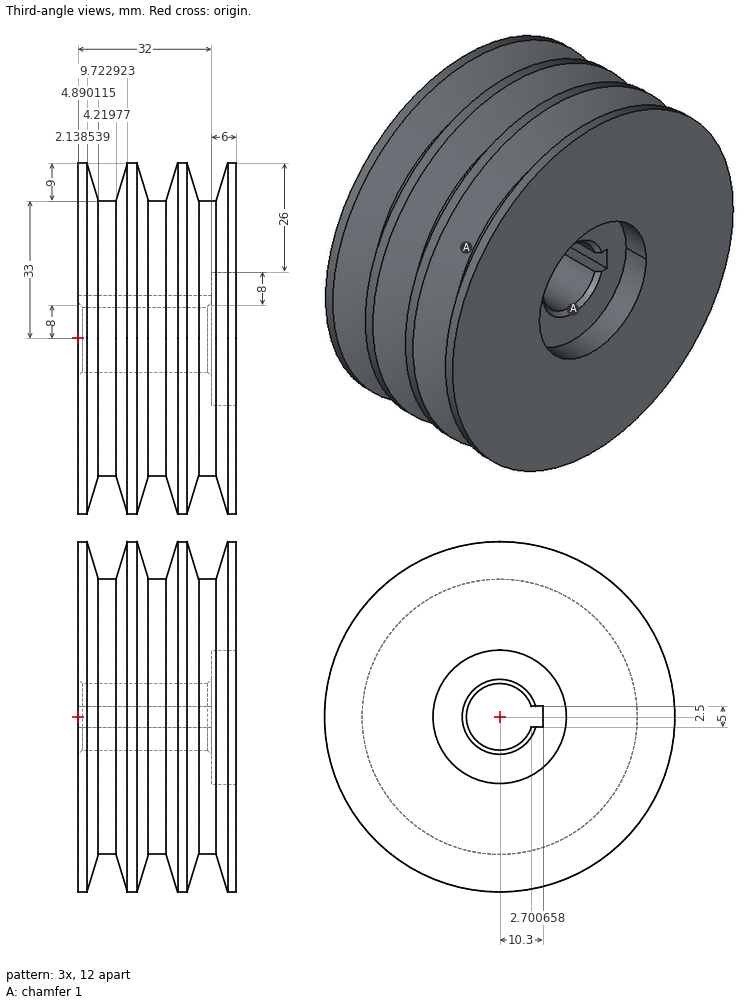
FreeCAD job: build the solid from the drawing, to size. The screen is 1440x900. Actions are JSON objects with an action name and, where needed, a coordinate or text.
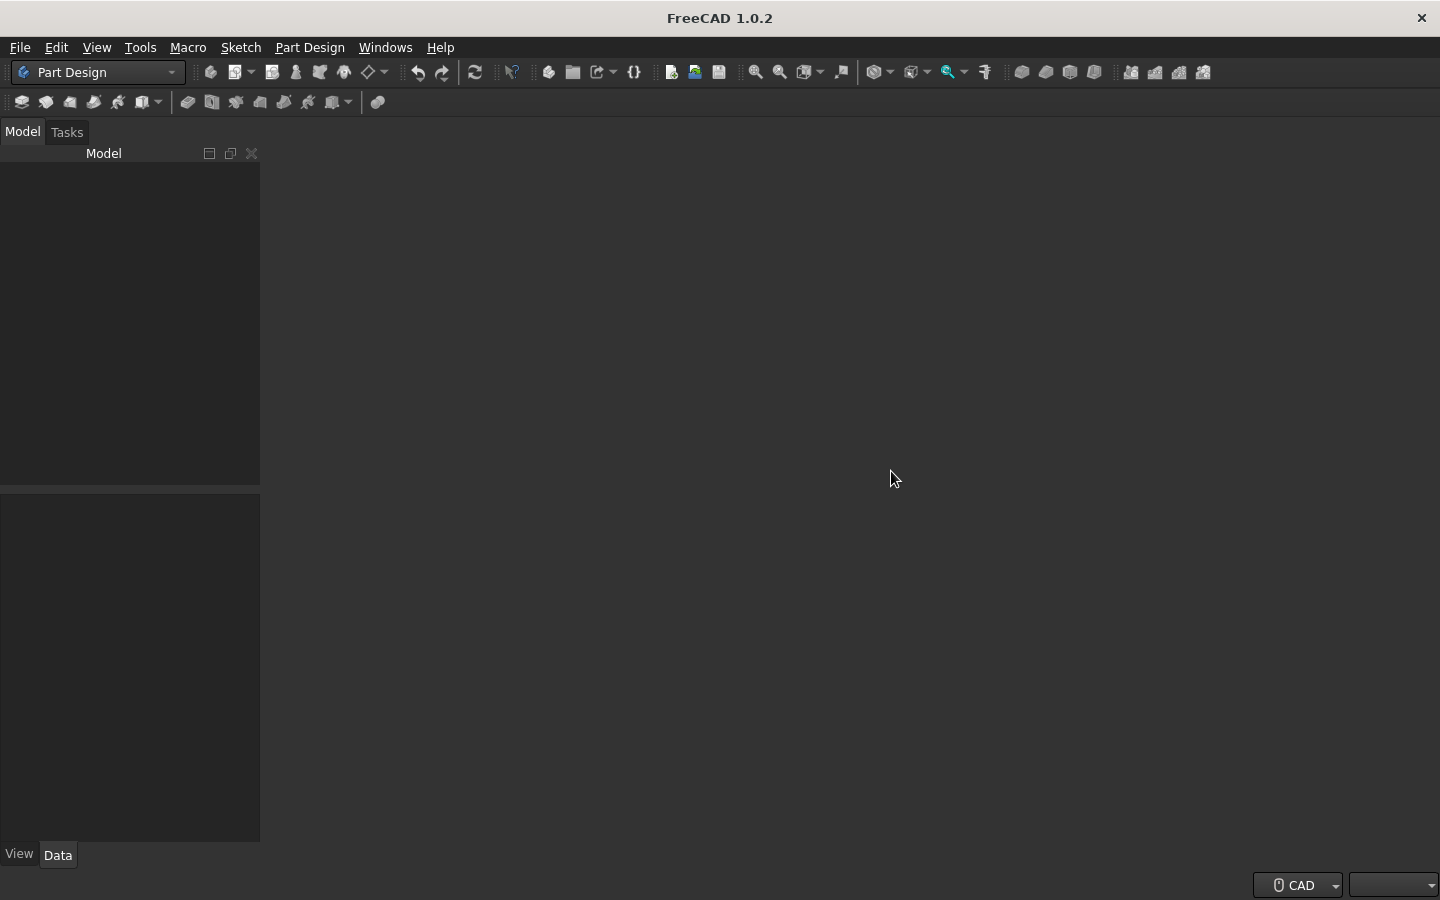
{"action": "key", "text": "ctrl+n"}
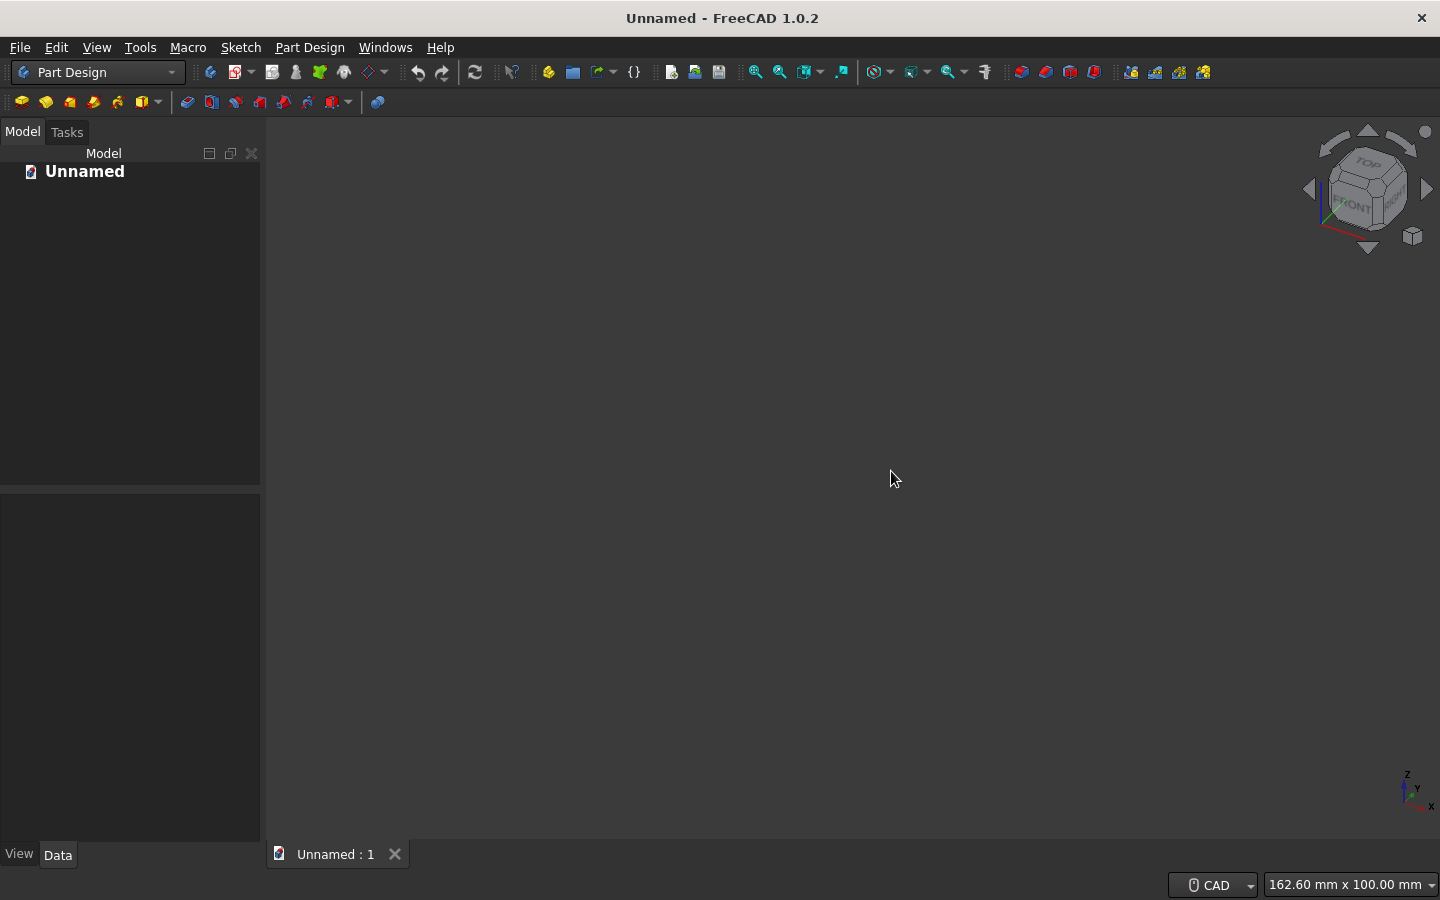
{"action": "left_click", "coordinate": [236, 72]}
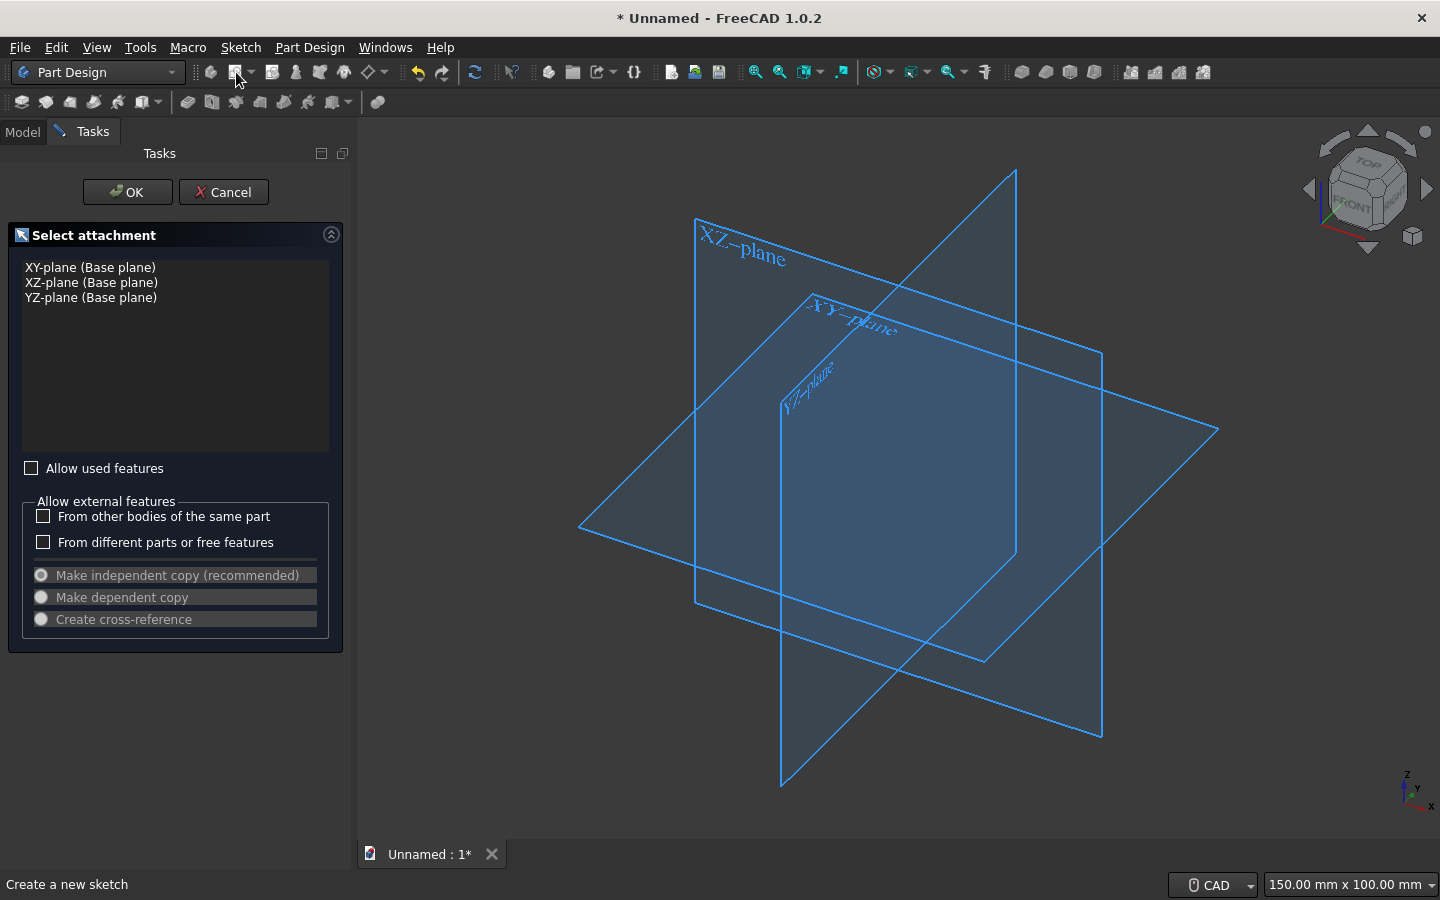
{"action": "left_click", "coordinate": [82, 268]}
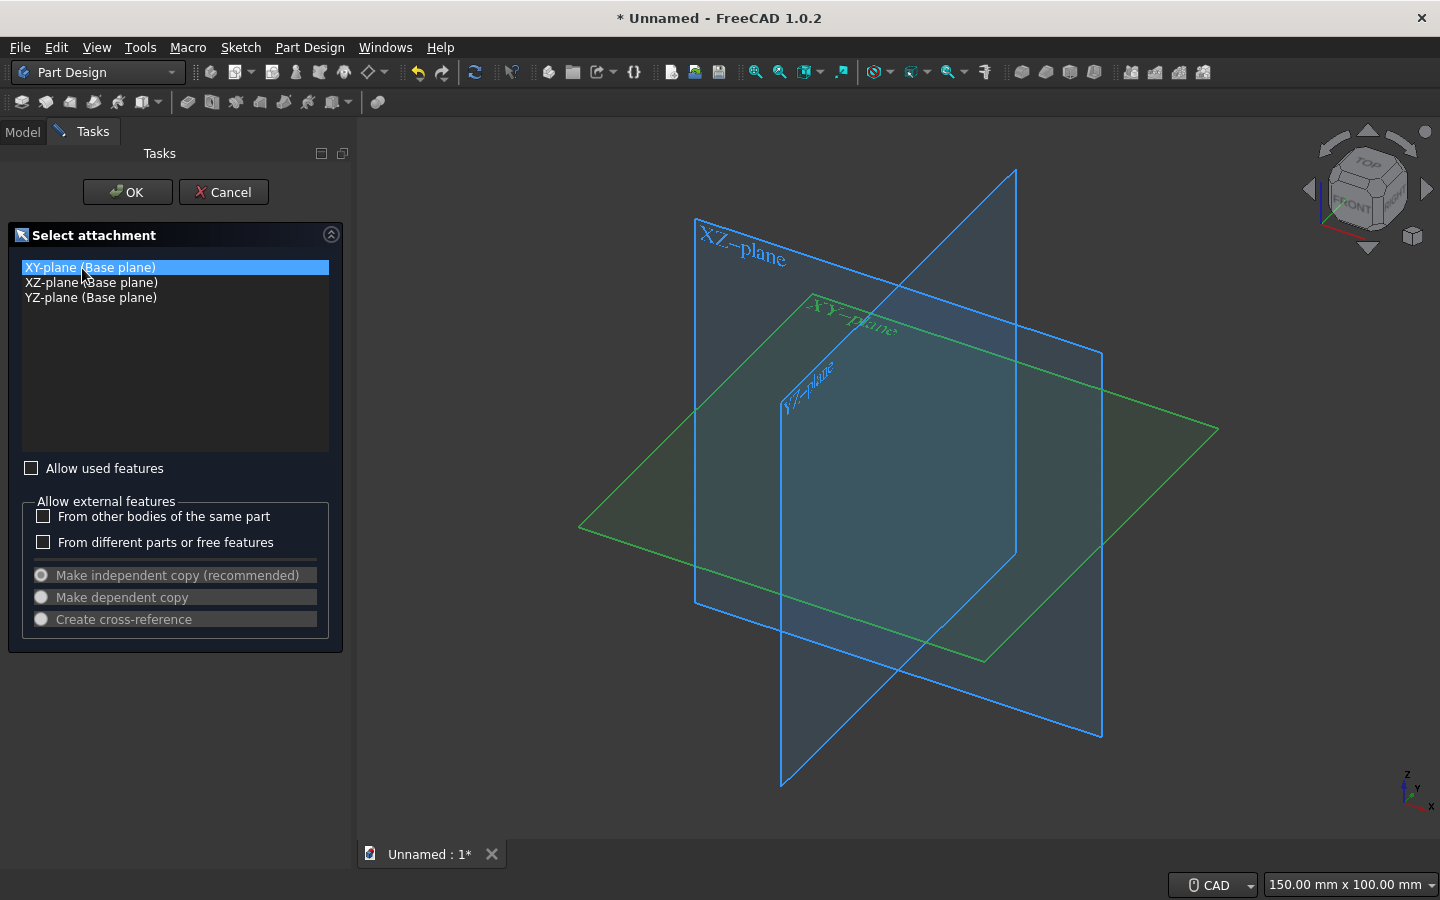
{"action": "left_click", "coordinate": [128, 192]}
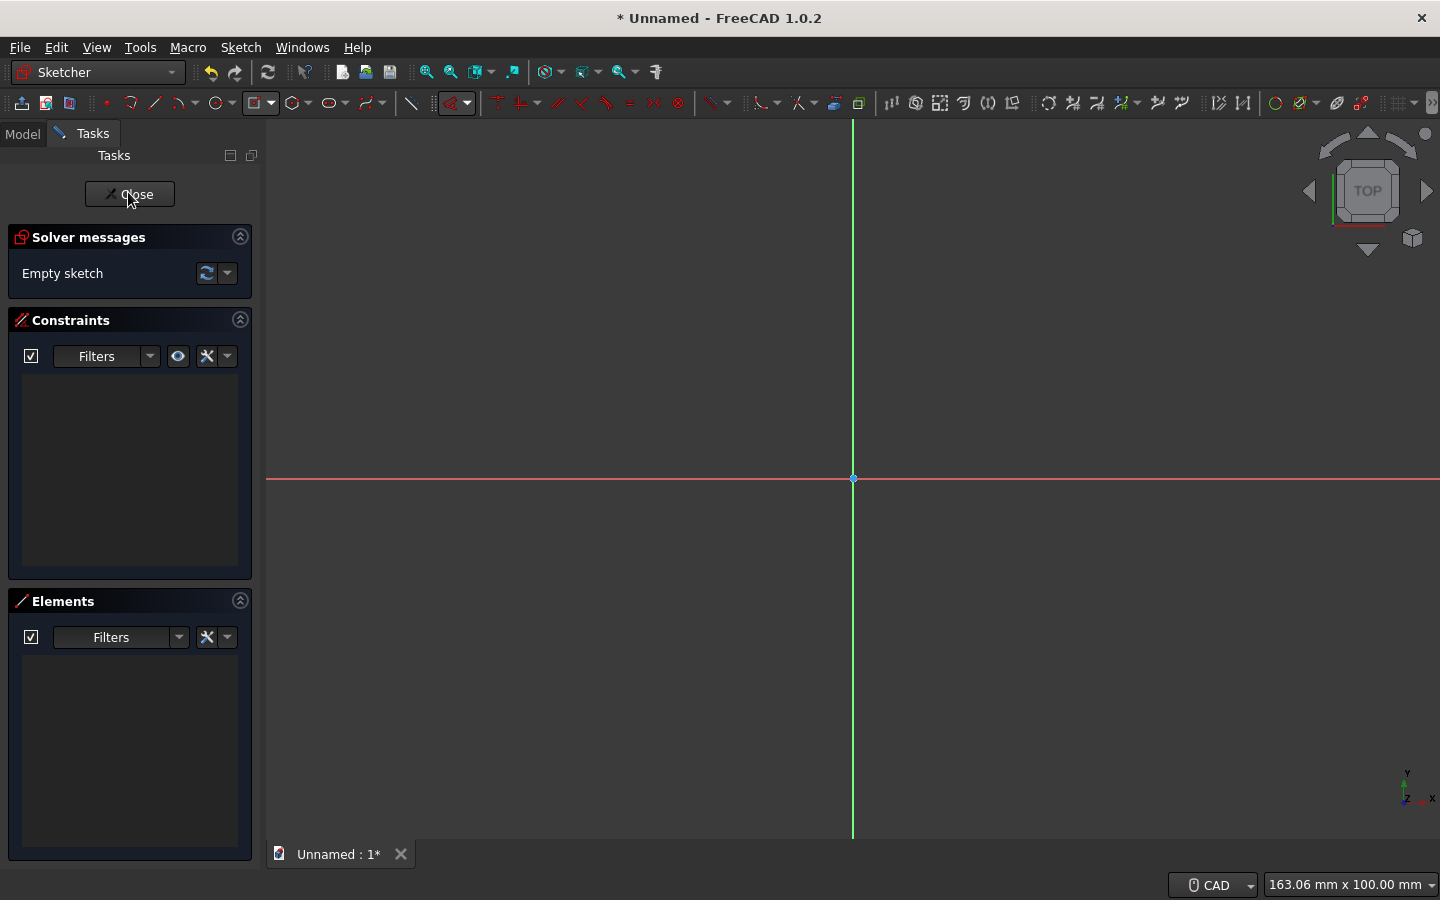
{"action": "scroll", "coordinate": [1275, 147], "scroll_direction": "up", "scroll_amount": 2}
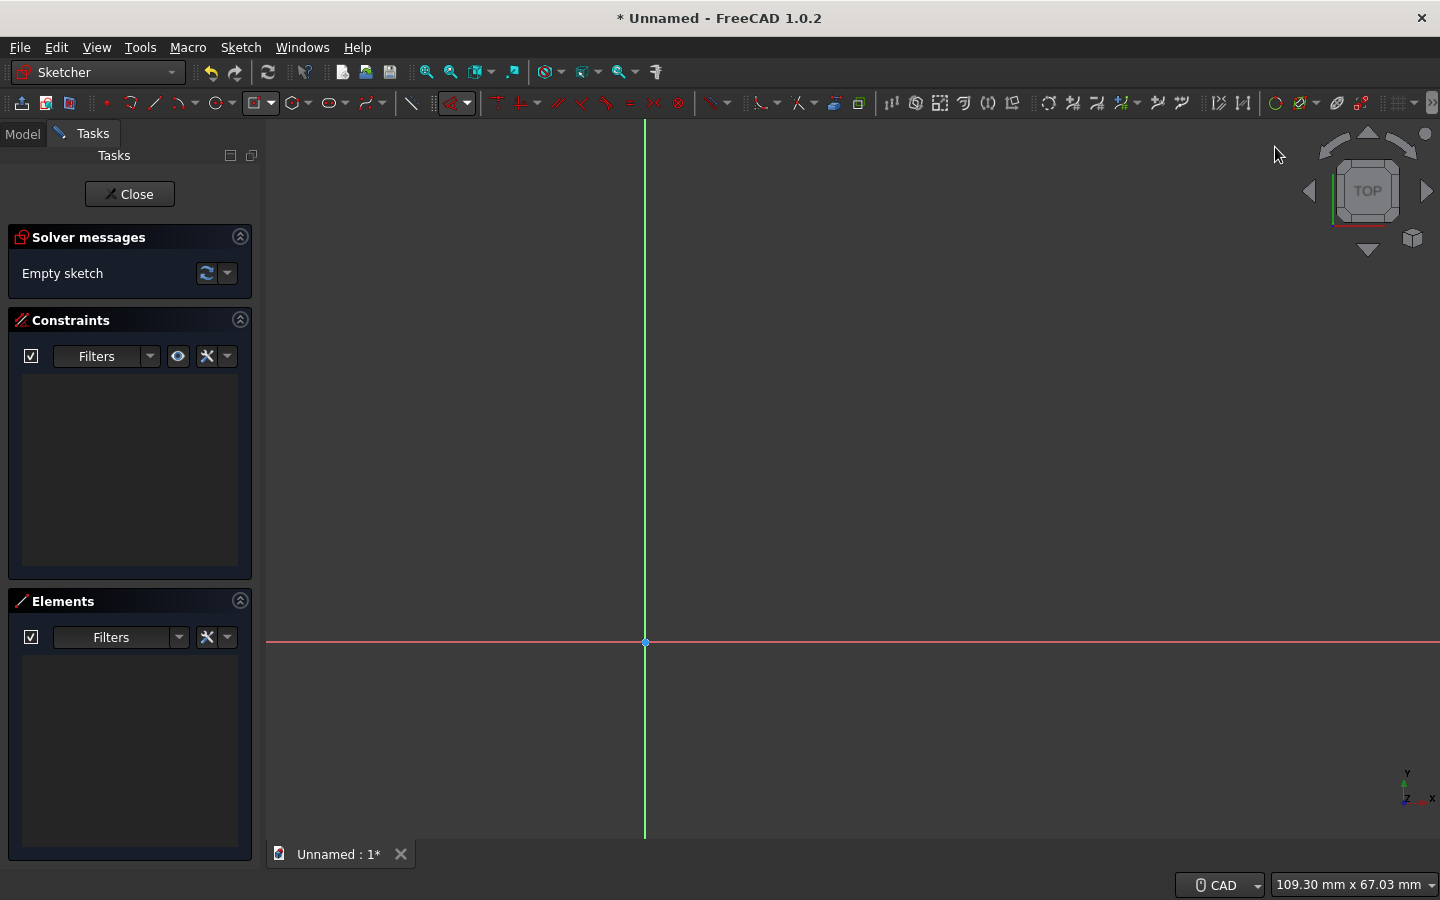
{"action": "key", "text": "g m"}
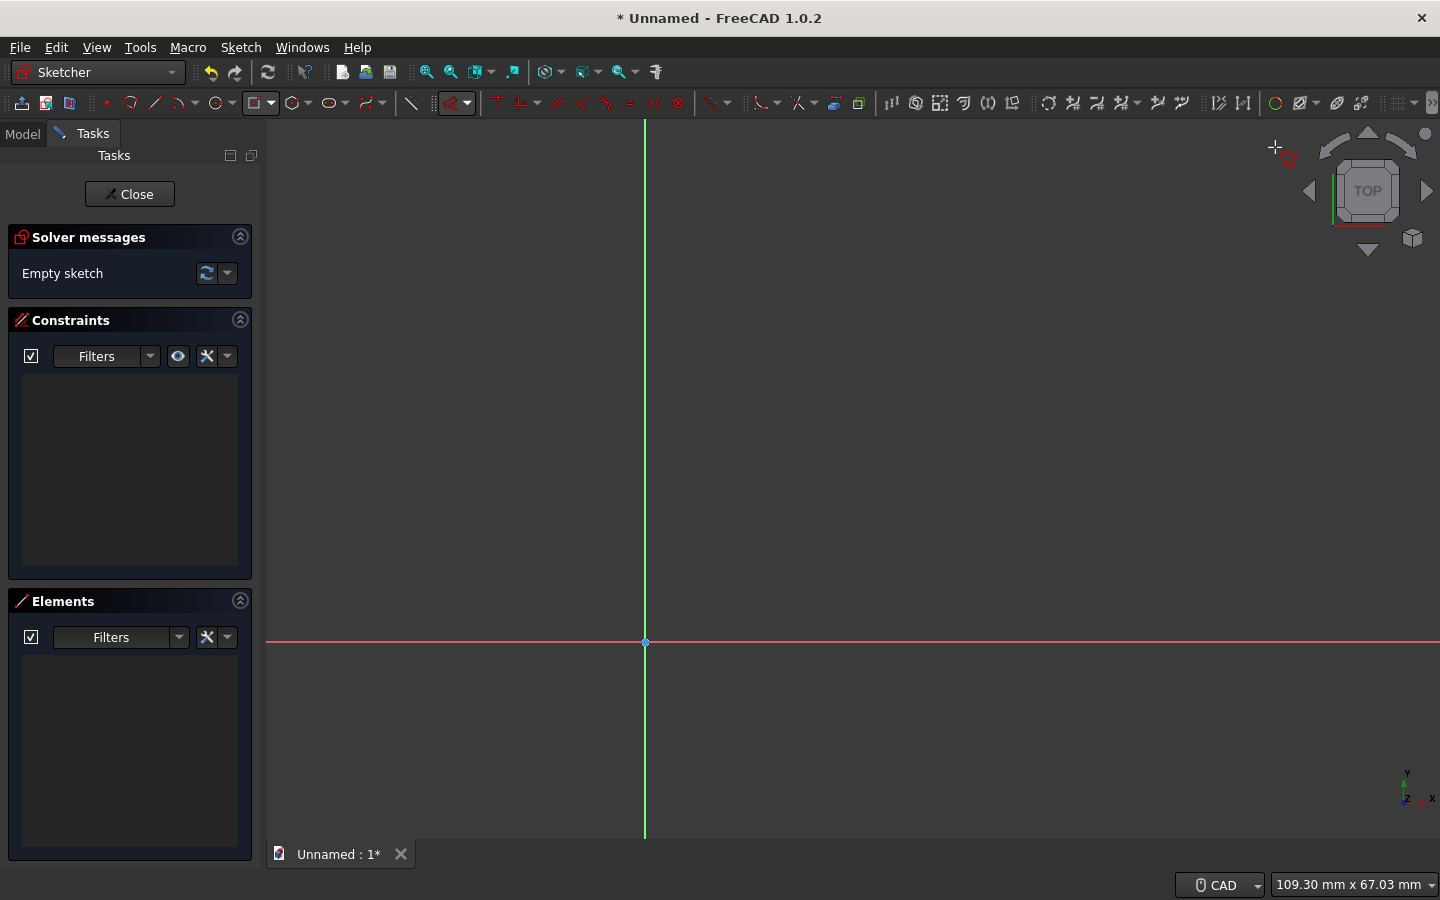
{"action": "left_click", "coordinate": [645, 556]}
{"action": "left_click", "coordinate": [989, 556]}
{"action": "left_click", "coordinate": [989, 470]}
{"action": "left_click", "coordinate": [1053, 470]}
{"action": "left_click", "coordinate": [1053, 191]}
{"action": "left_click", "coordinate": [654, 191]}
{"action": "left_click", "coordinate": [645, 557]}
{"action": "key", "text": "Escape"}
{"action": "key", "text": "Escape"}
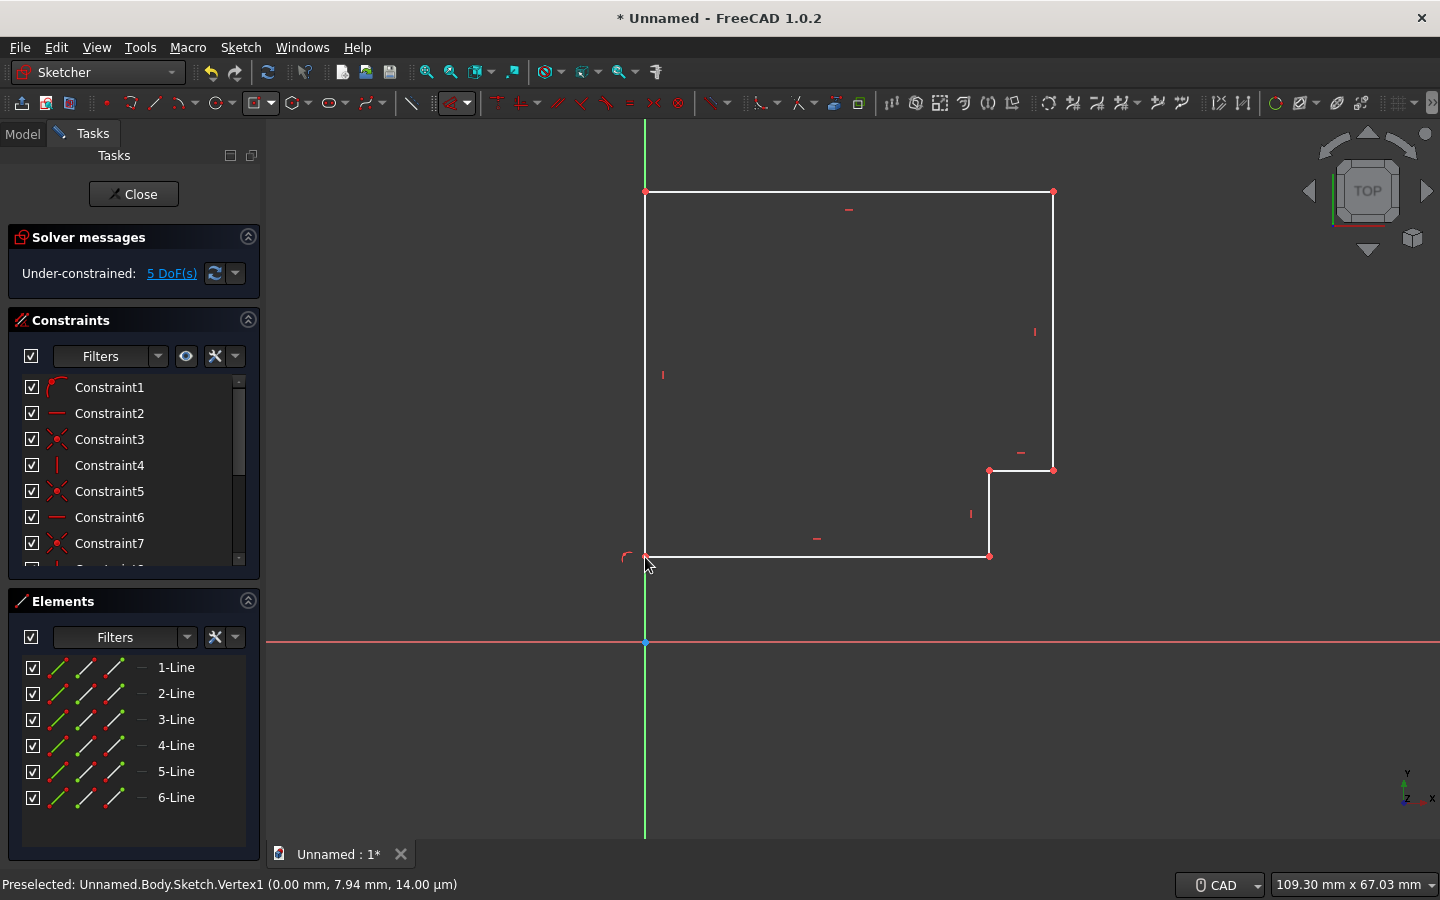
{"action": "key", "text": "d"}